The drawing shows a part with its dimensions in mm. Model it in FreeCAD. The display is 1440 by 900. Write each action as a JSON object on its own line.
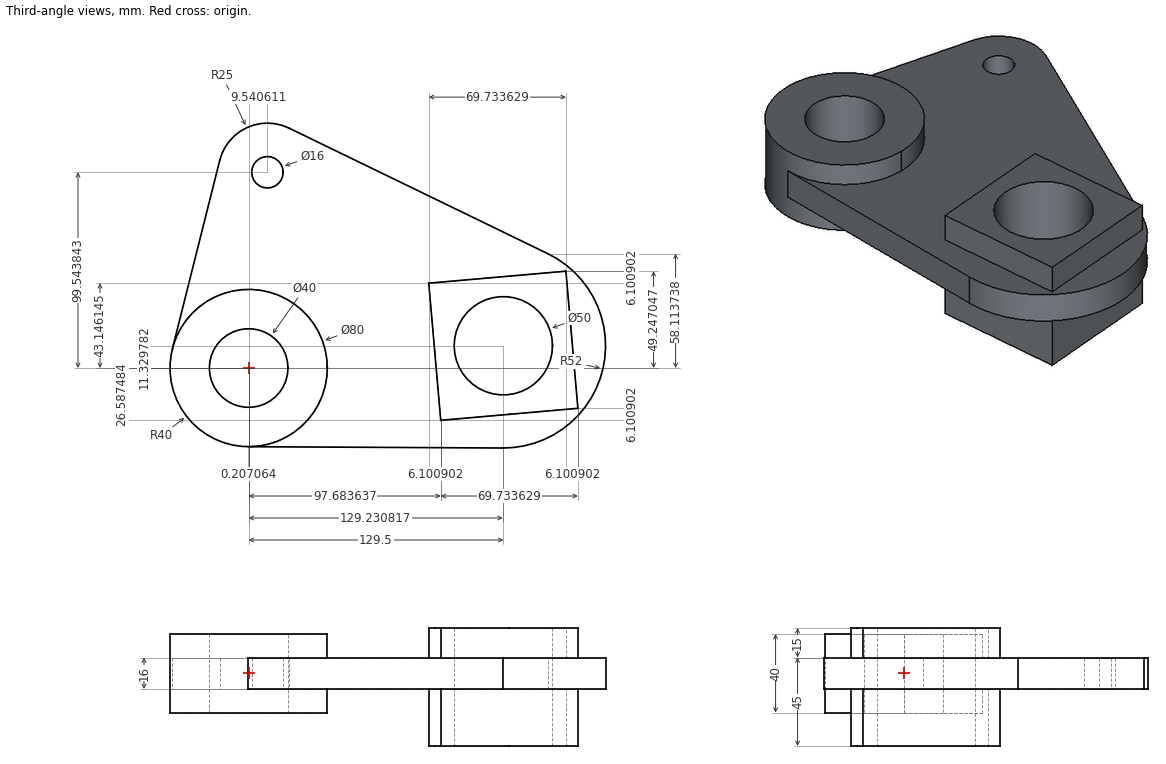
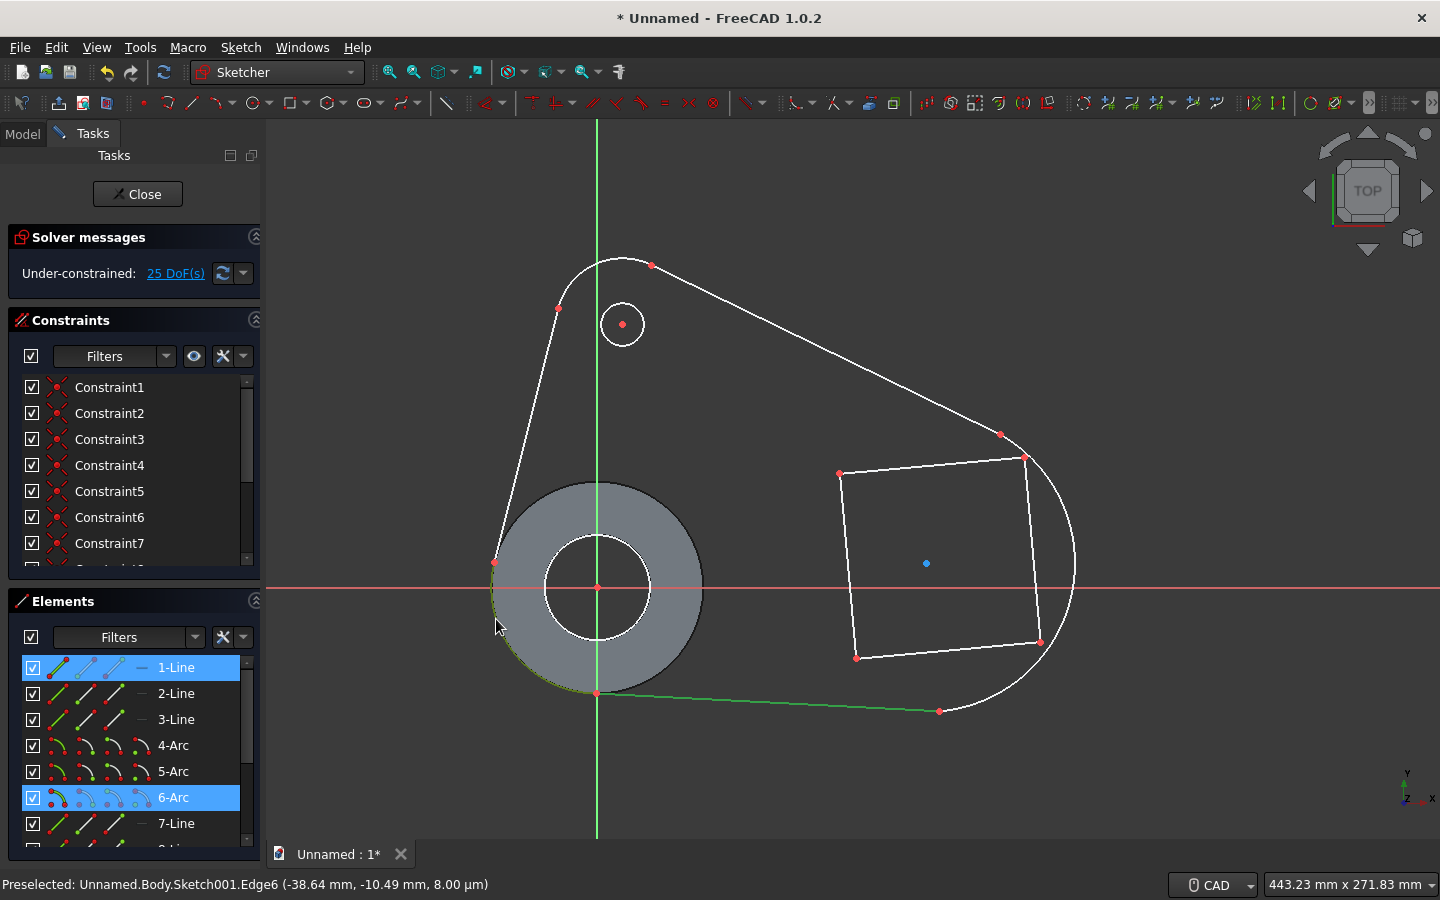
{"action": "key", "text": "t"}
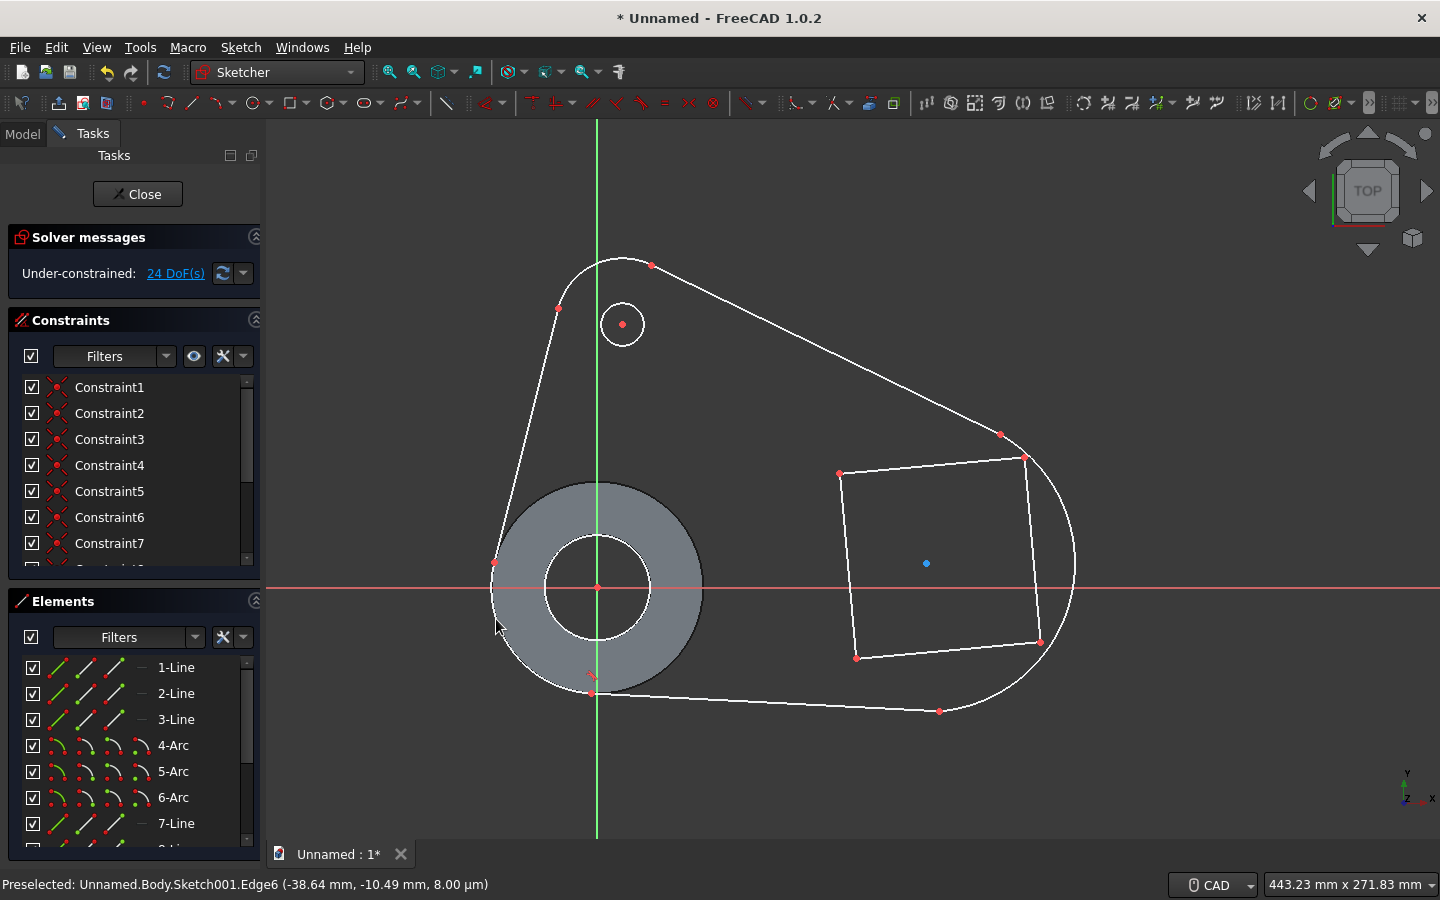
{"action": "left_click", "coordinate": [896, 384]}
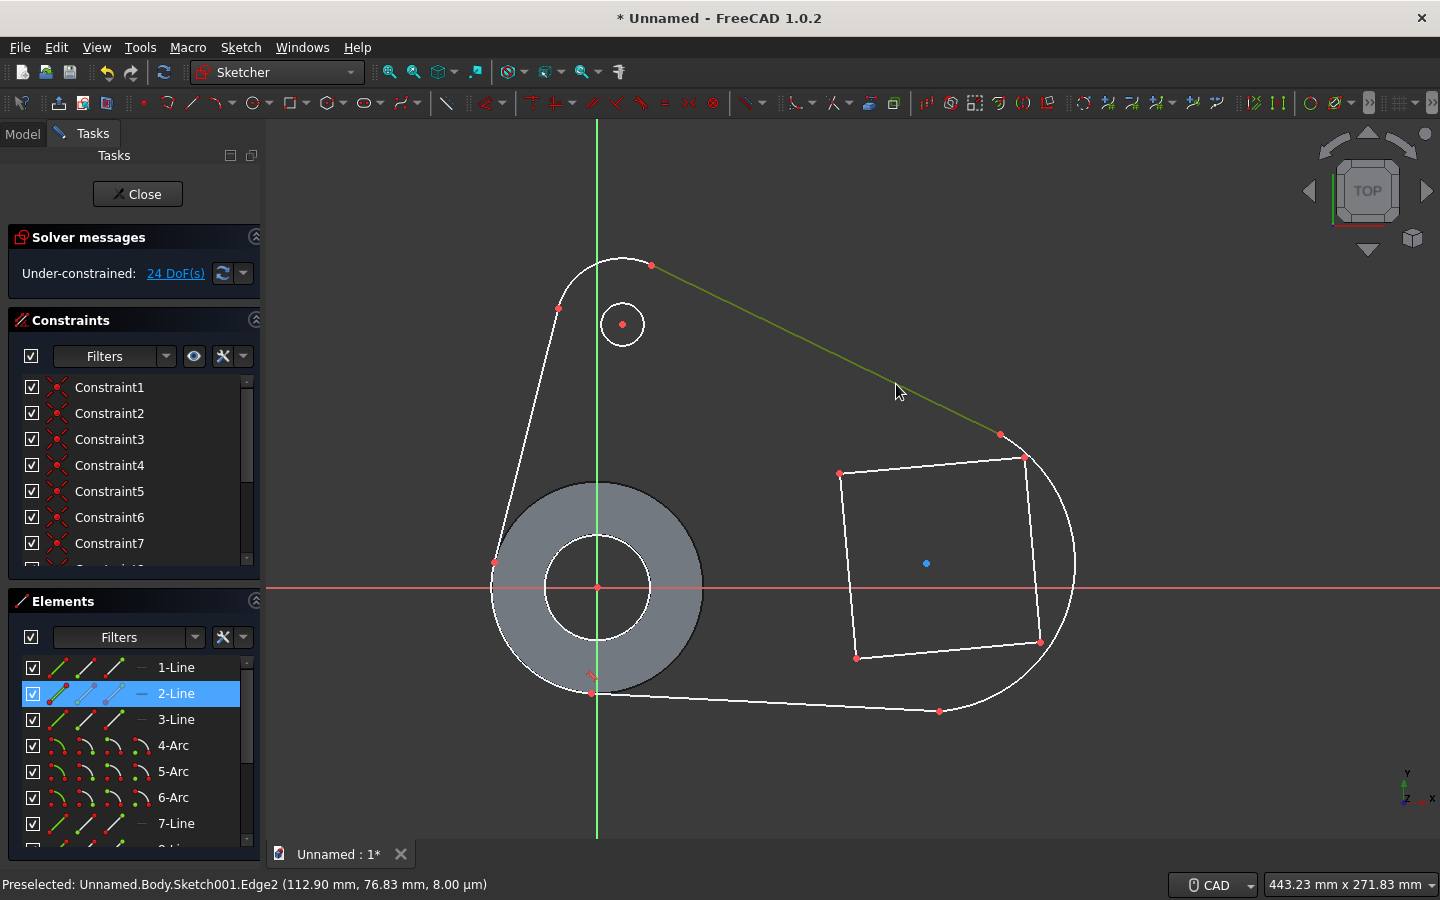
{"action": "left_click", "coordinate": [617, 259]}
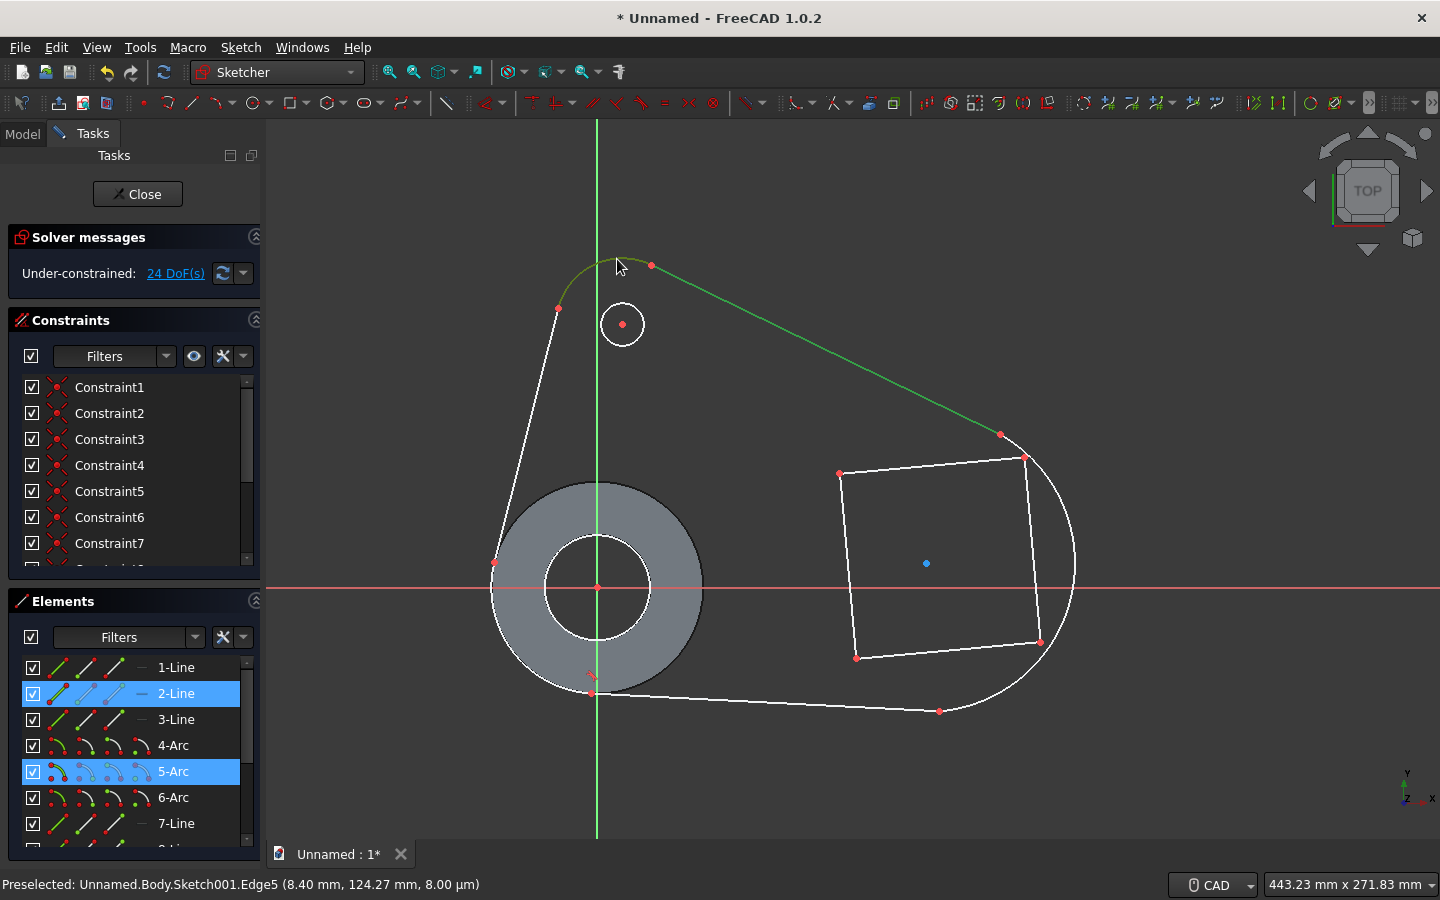
{"action": "key", "text": "t"}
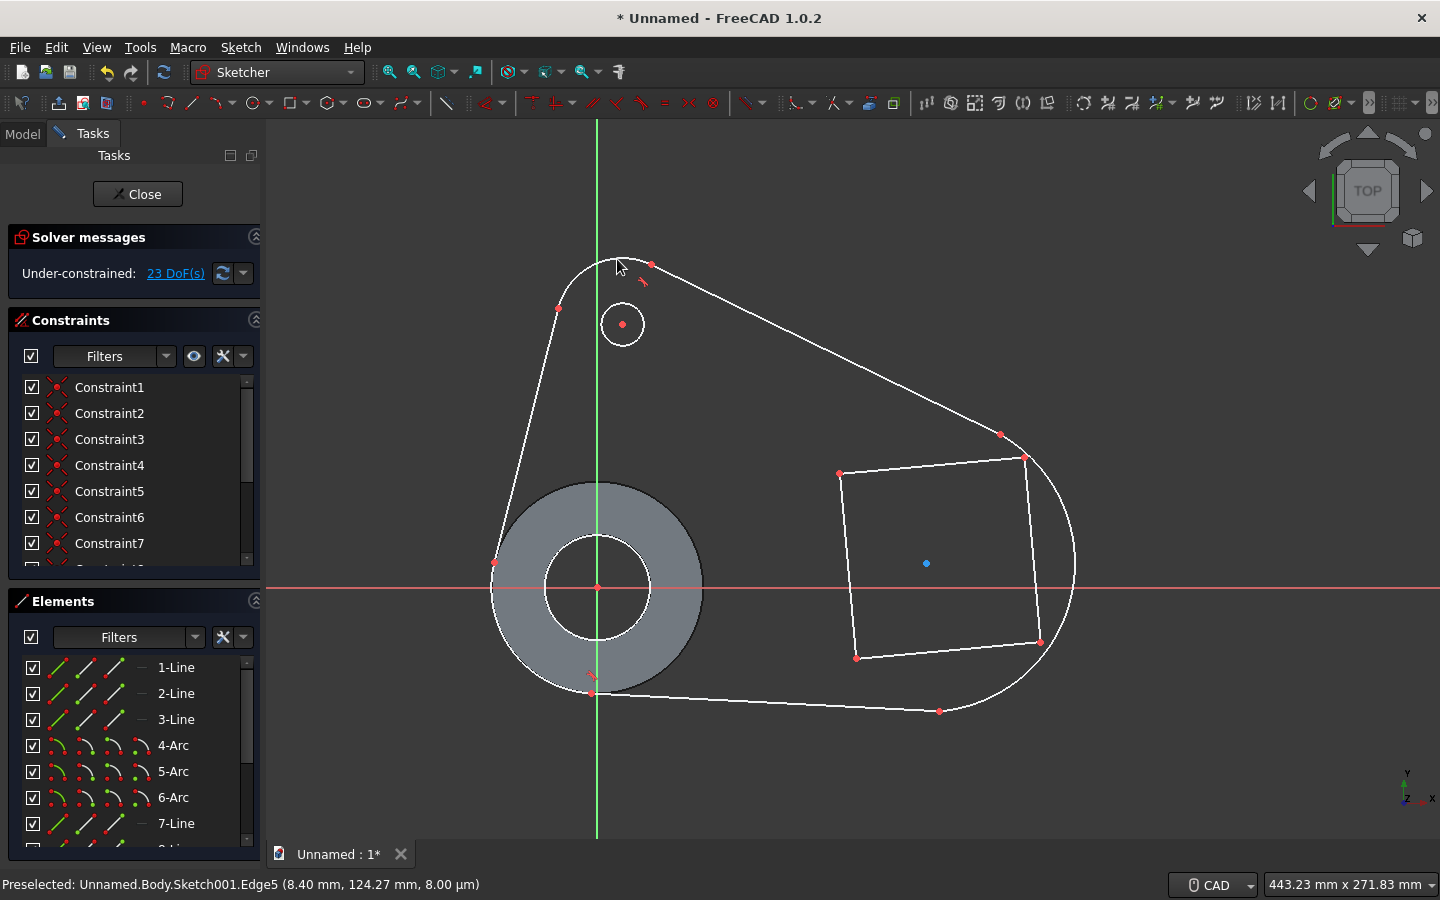
{"action": "left_click", "coordinate": [539, 385]}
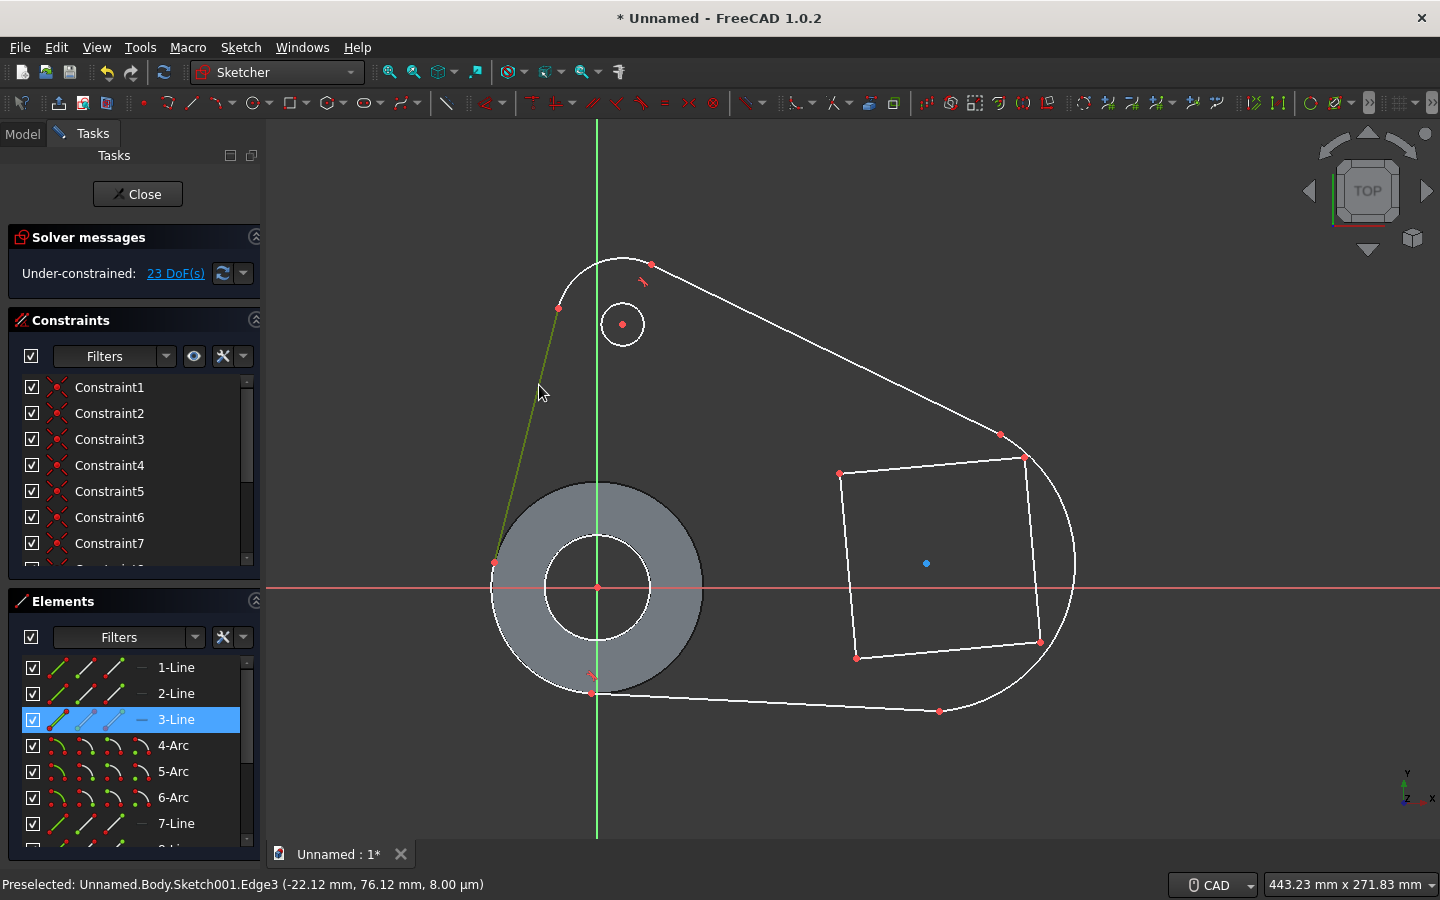
{"action": "left_click", "coordinate": [617, 258]}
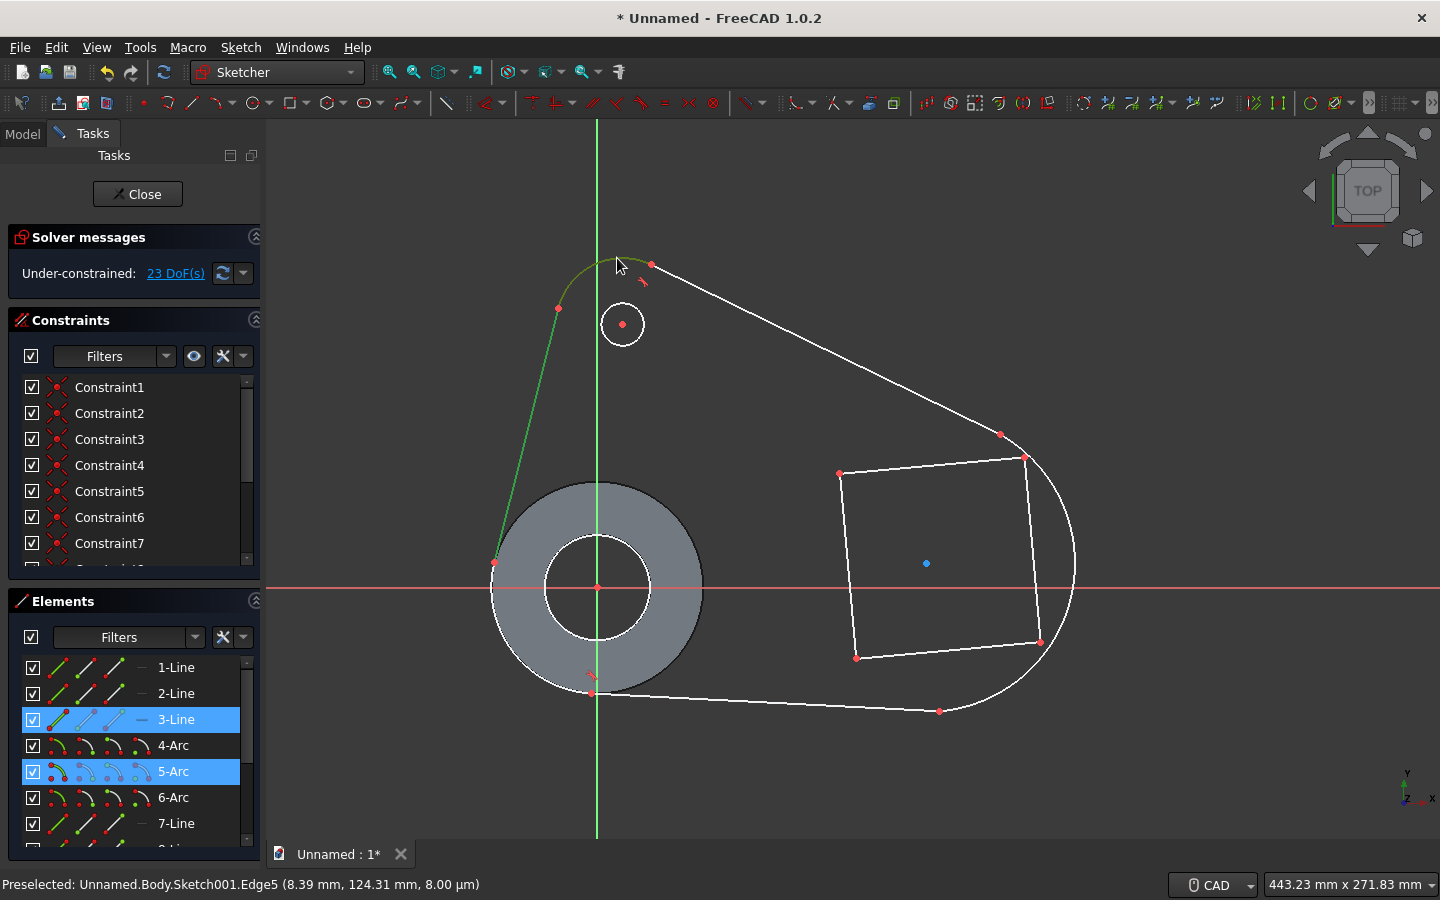
{"action": "key", "text": "t"}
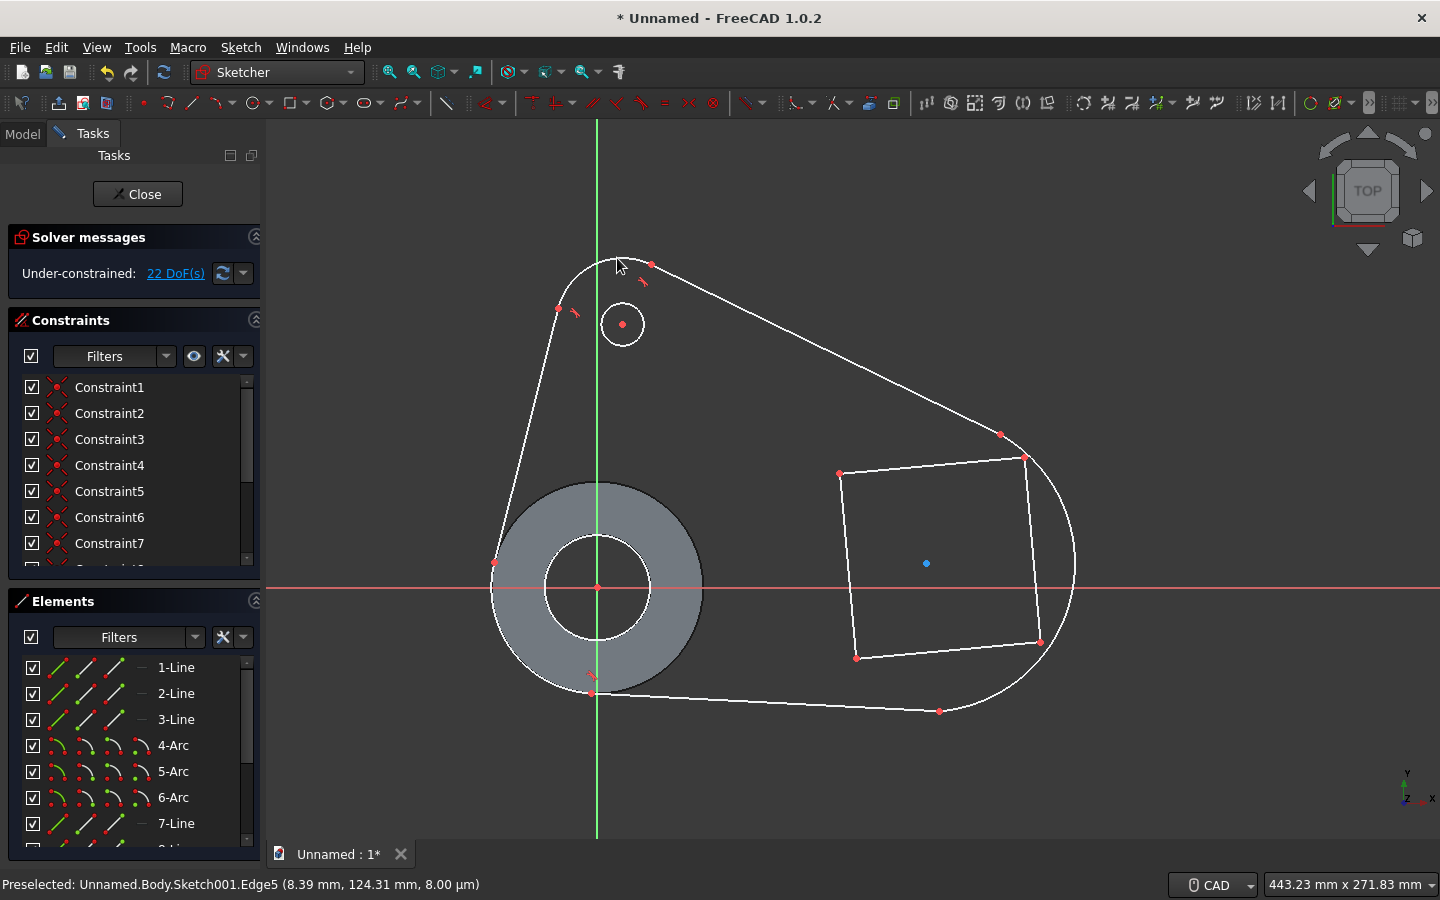
{"action": "left_click", "coordinate": [539, 385]}